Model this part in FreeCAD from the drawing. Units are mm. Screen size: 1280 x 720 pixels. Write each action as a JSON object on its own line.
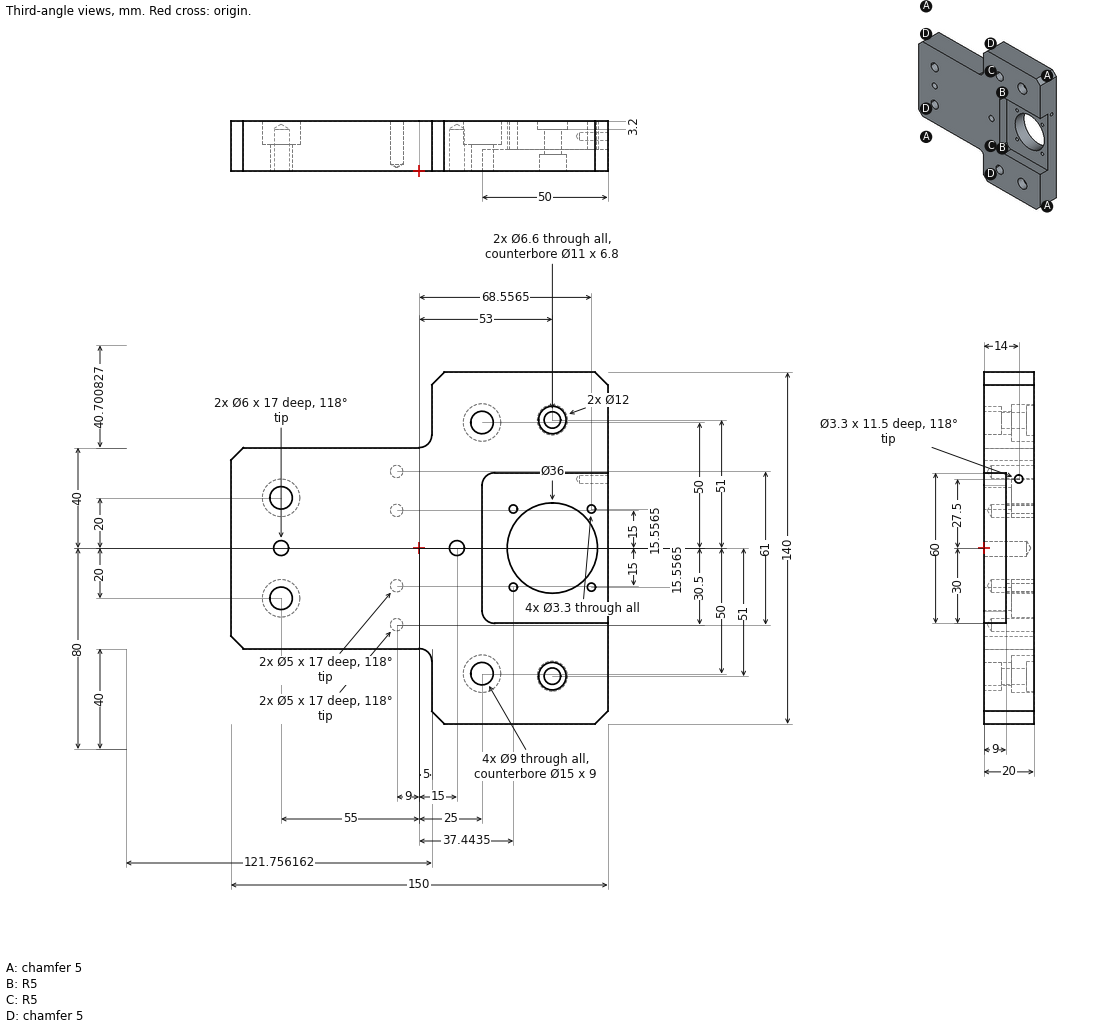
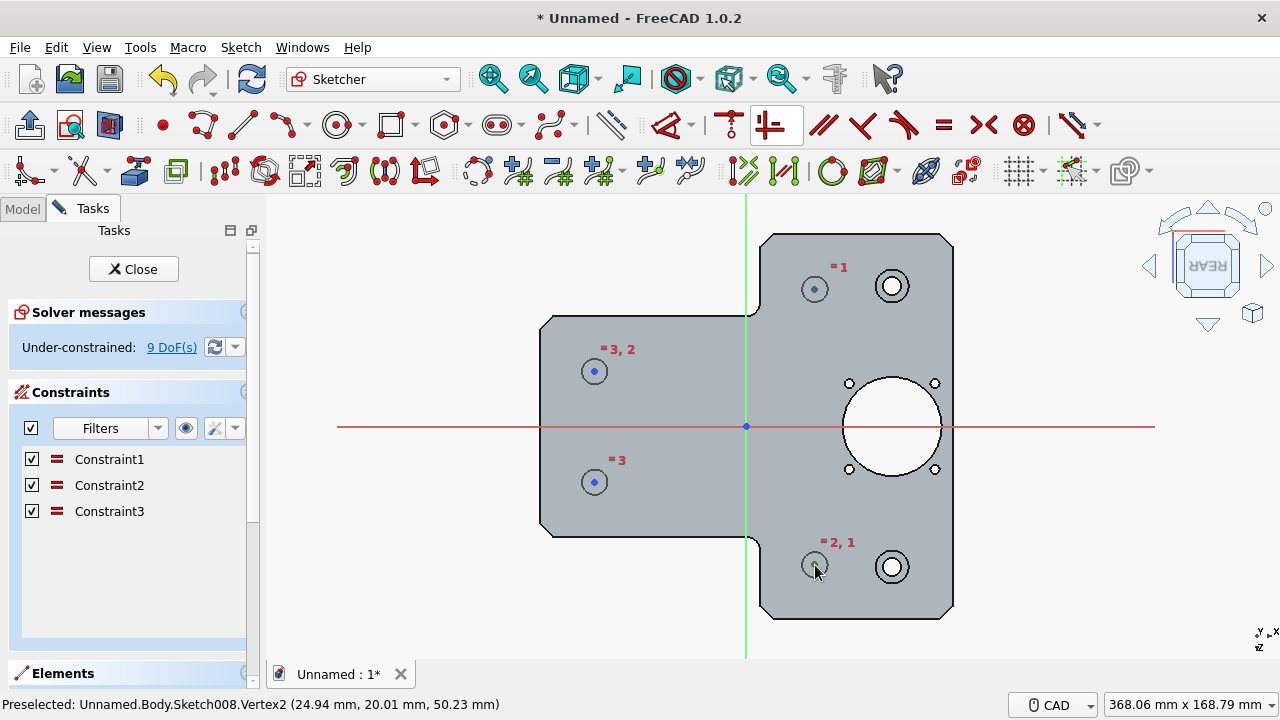
{"action": "key", "text": "v"}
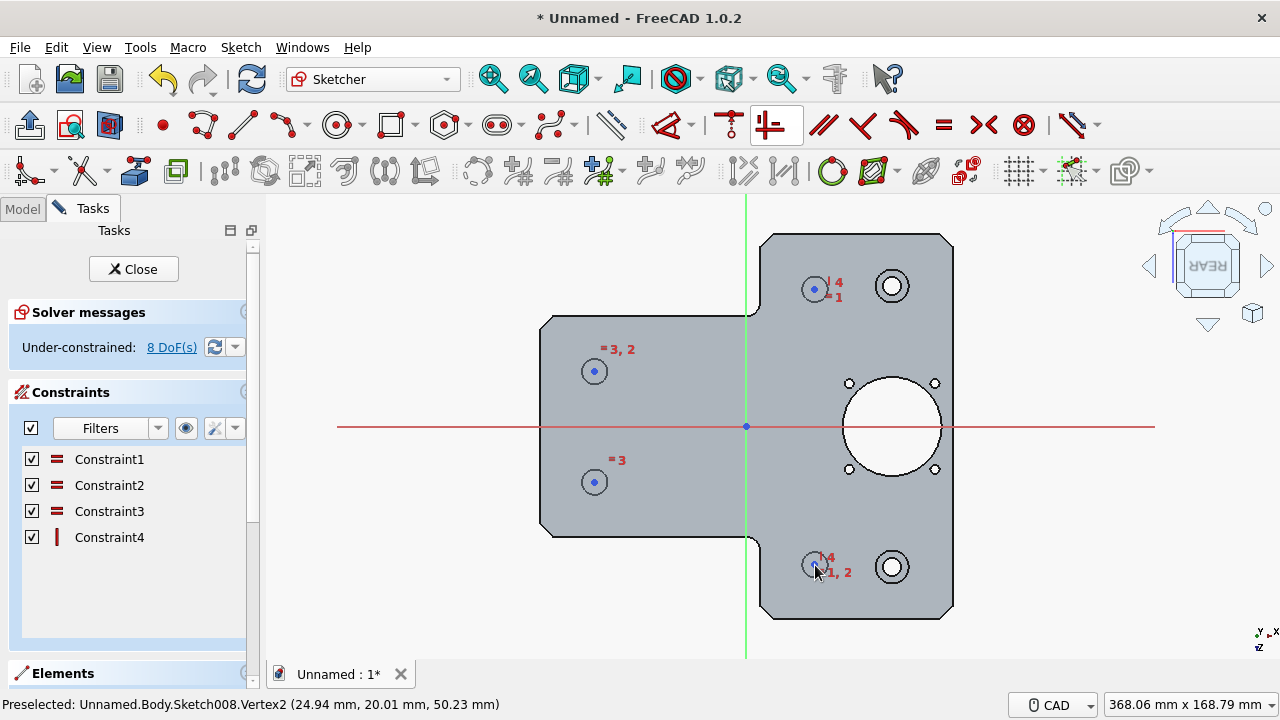
{"action": "left_click", "coordinate": [595, 372]}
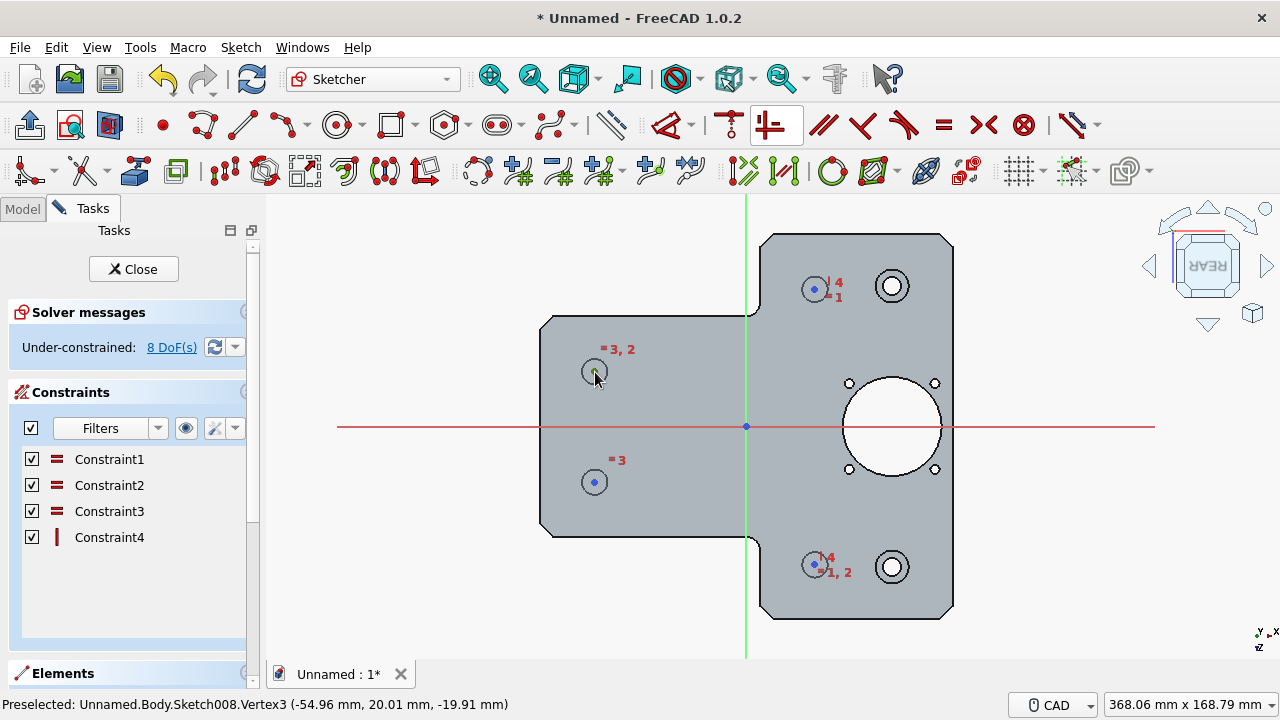
{"action": "left_click", "coordinate": [595, 482]}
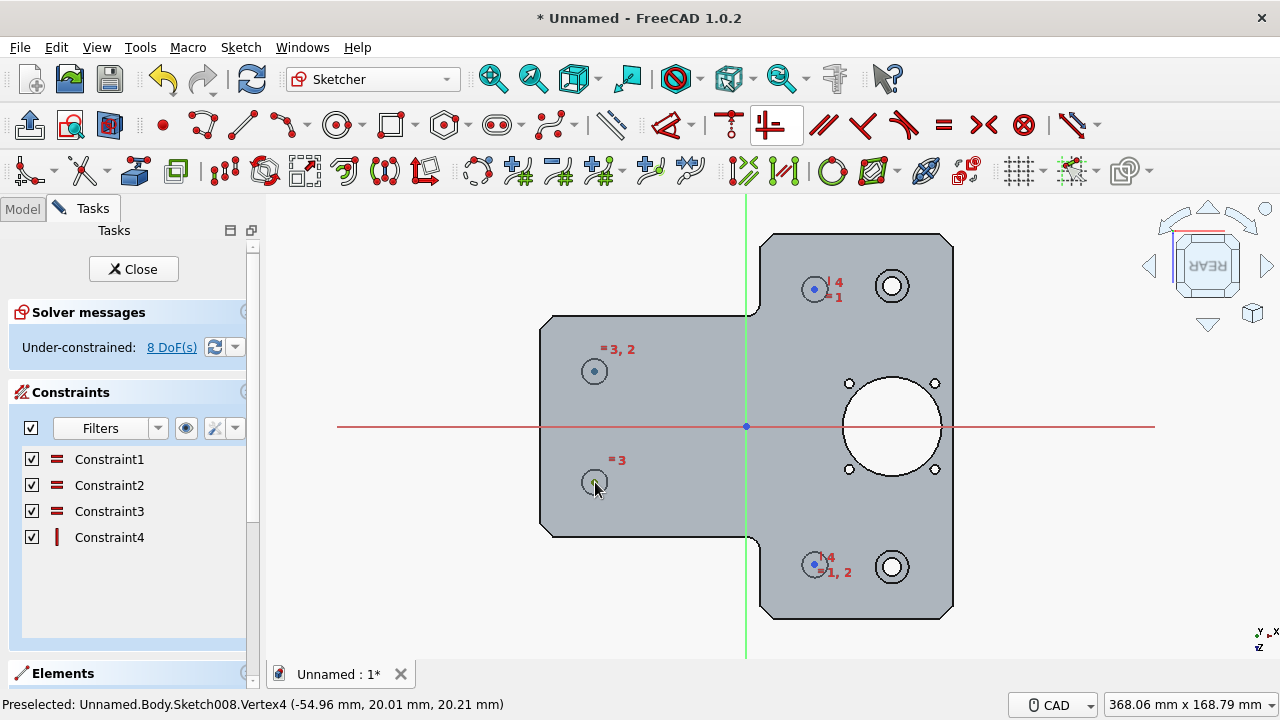
{"action": "left_click", "coordinate": [798, 126]}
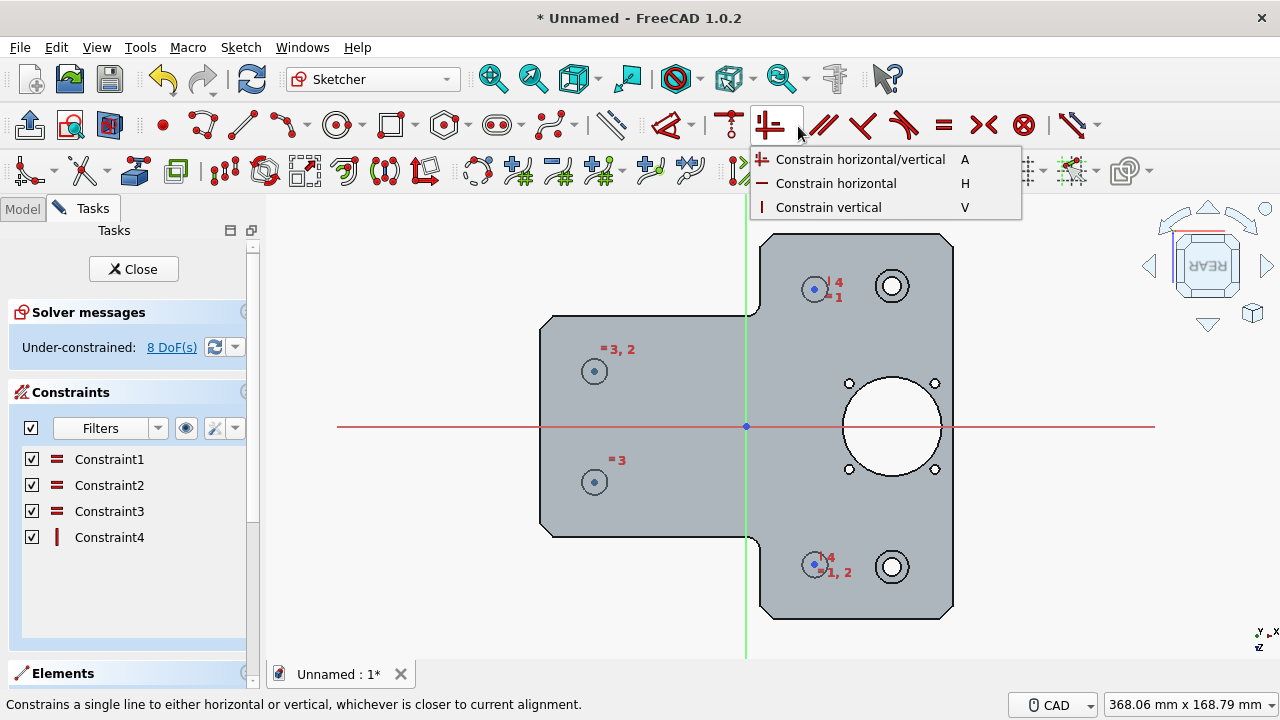
{"action": "left_click", "coordinate": [886, 207]}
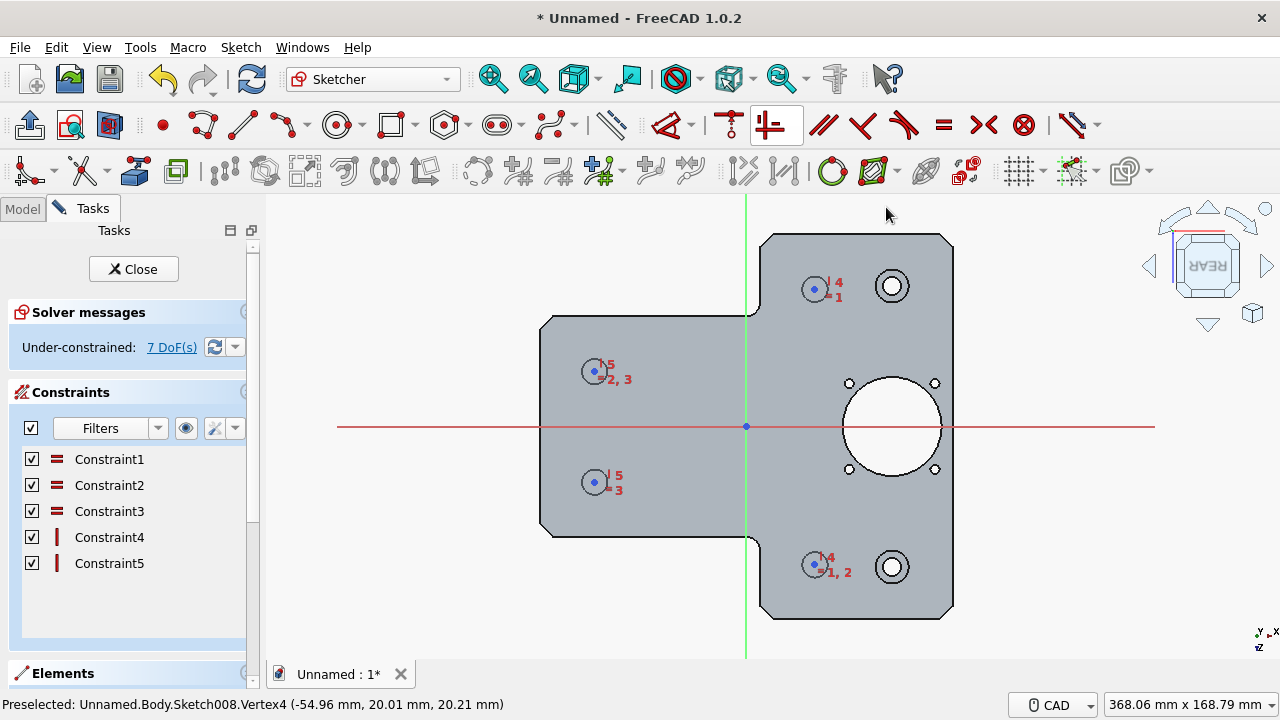
{"action": "left_click", "coordinate": [666, 126]}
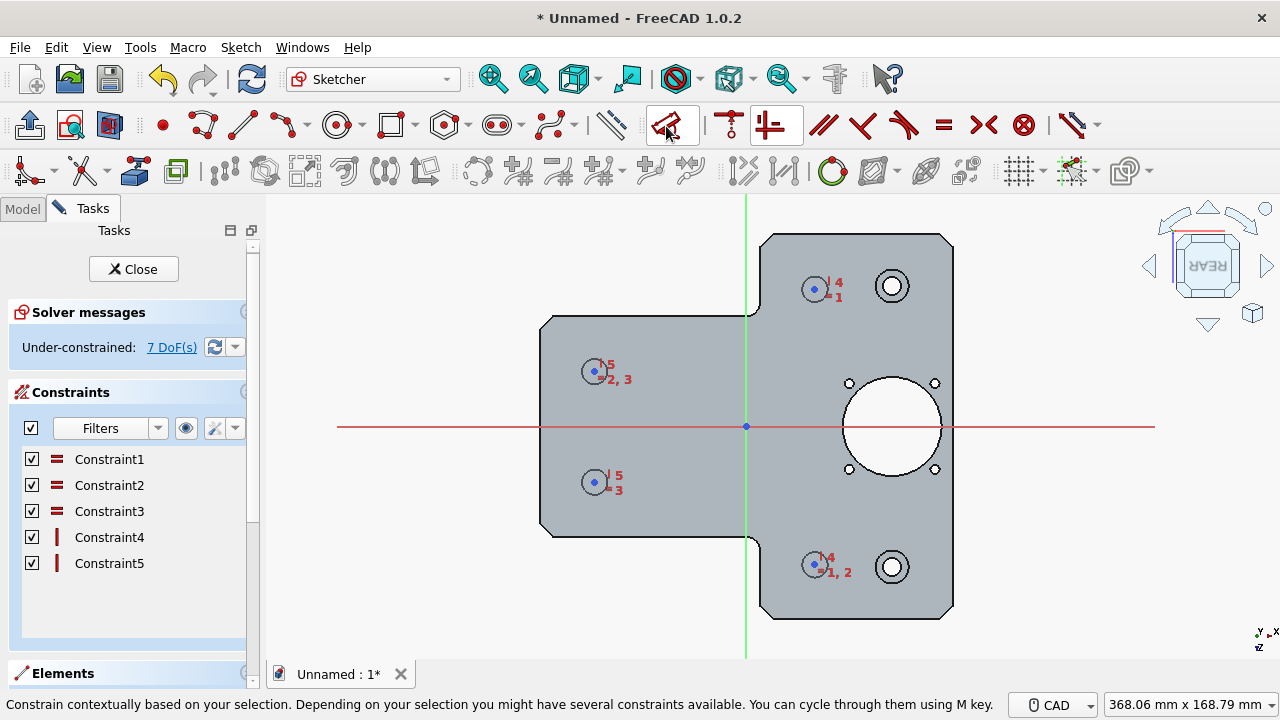
{"action": "scroll", "coordinate": [824, 280], "scroll_direction": "up", "scroll_amount": 3}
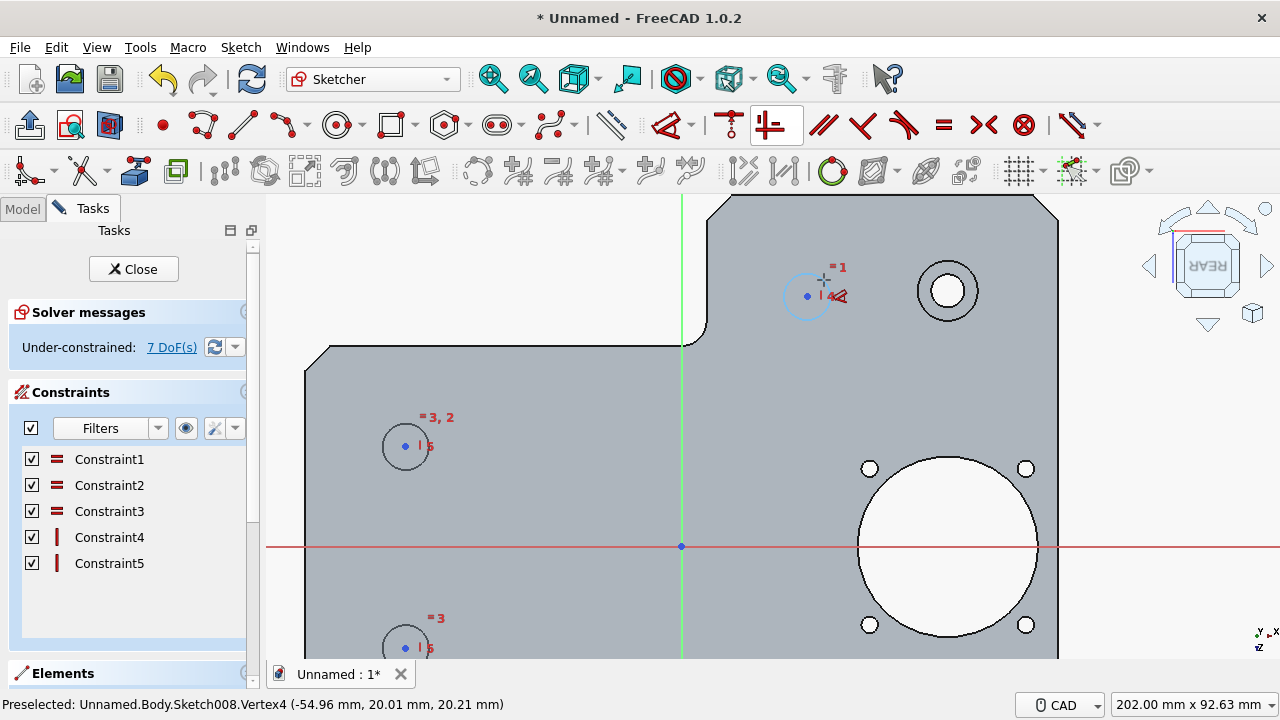
{"action": "left_click", "coordinate": [823, 280]}
{"action": "left_click", "coordinate": [845, 257]}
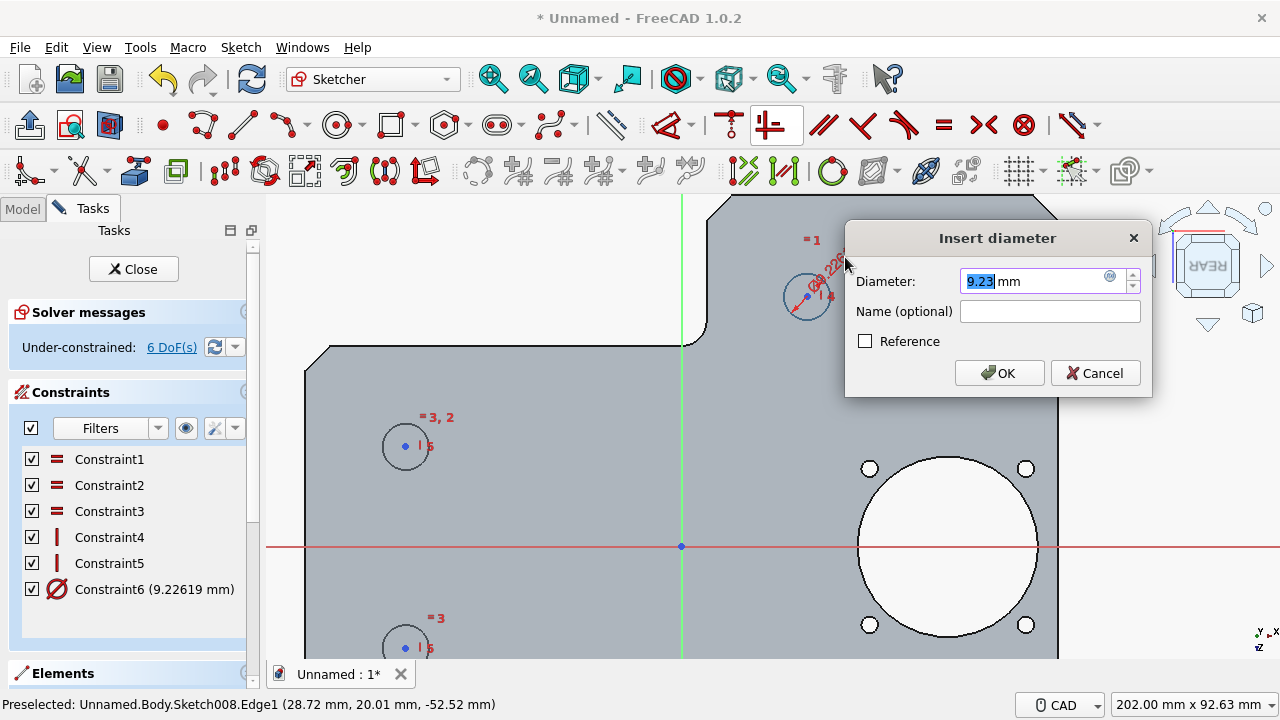
{"action": "type", "text": "9"}
{"action": "key", "text": "Return"}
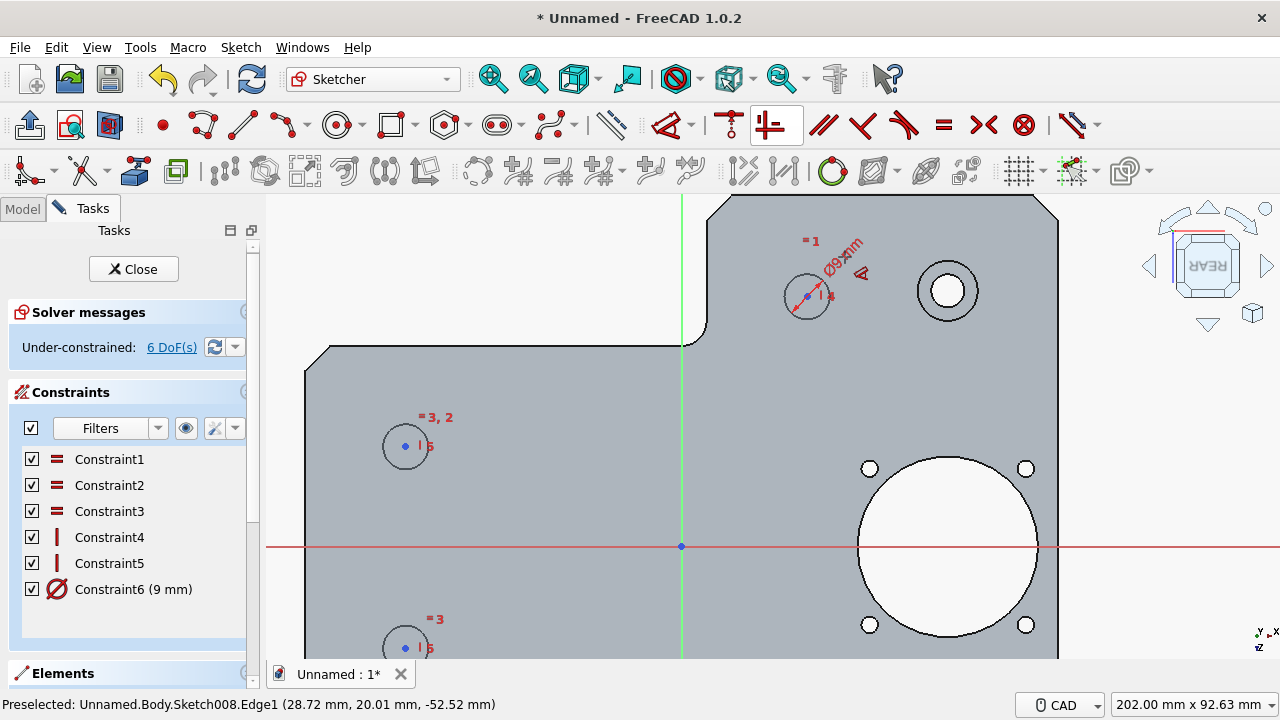
{"action": "left_click", "coordinate": [807, 297]}
{"action": "left_click", "coordinate": [744, 263]}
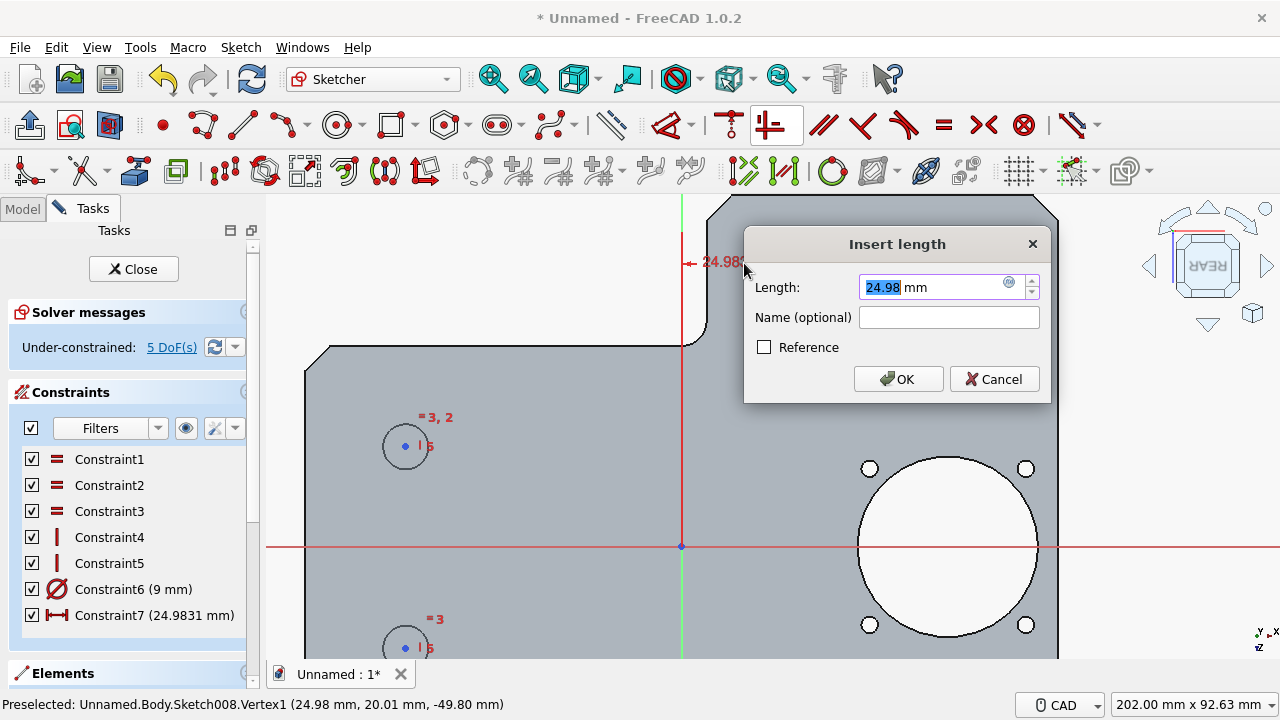
{"action": "type", "text": "25"}
{"action": "key", "text": "Return"}